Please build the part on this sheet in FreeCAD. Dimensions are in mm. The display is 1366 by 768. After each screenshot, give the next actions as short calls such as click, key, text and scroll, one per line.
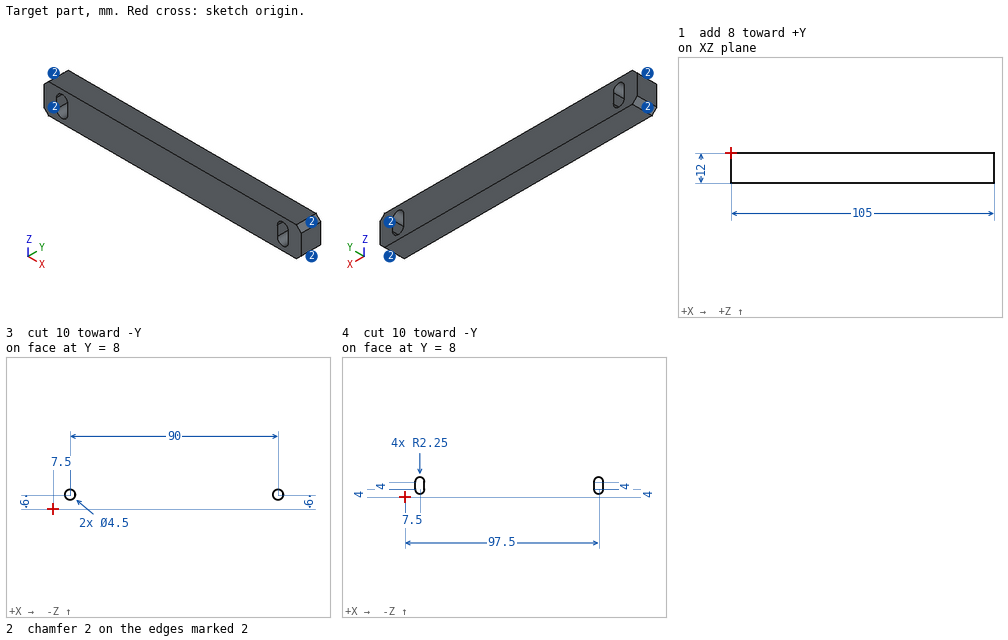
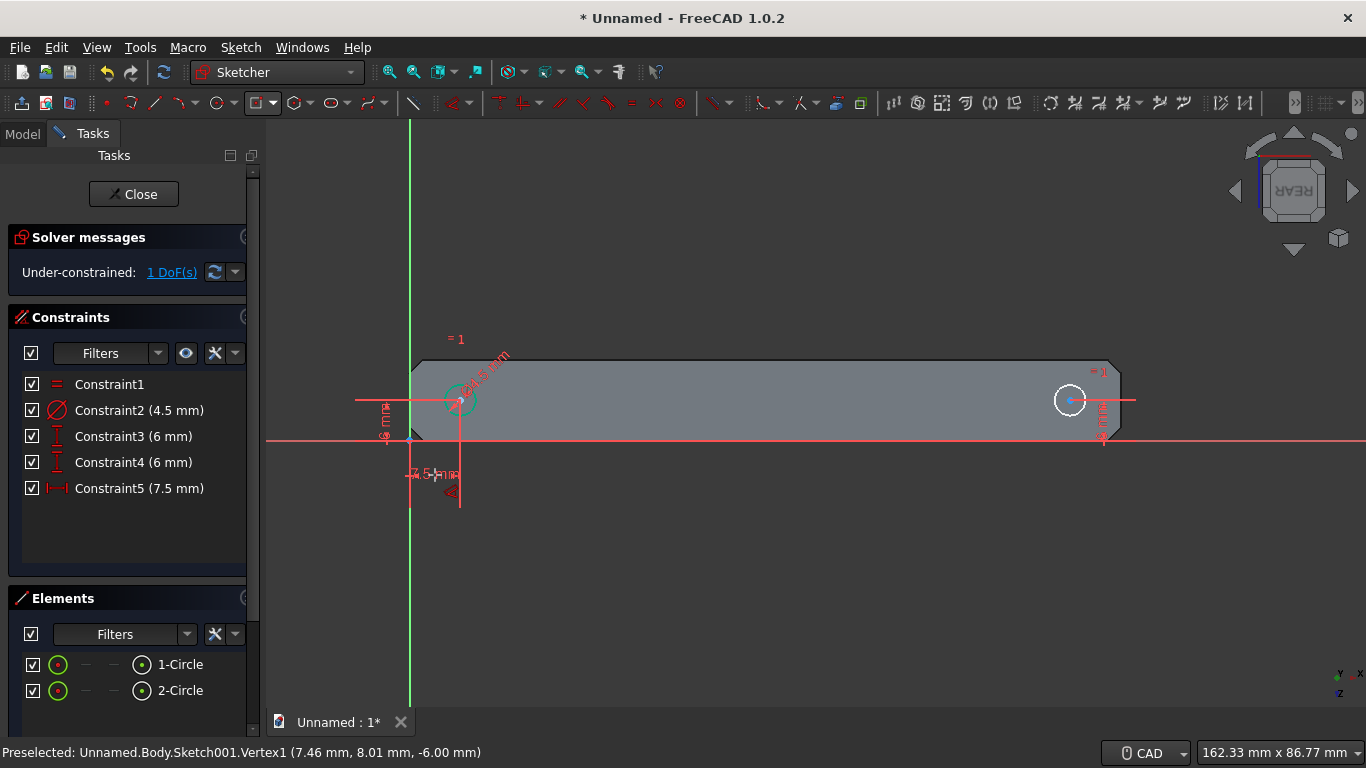
click(460, 400)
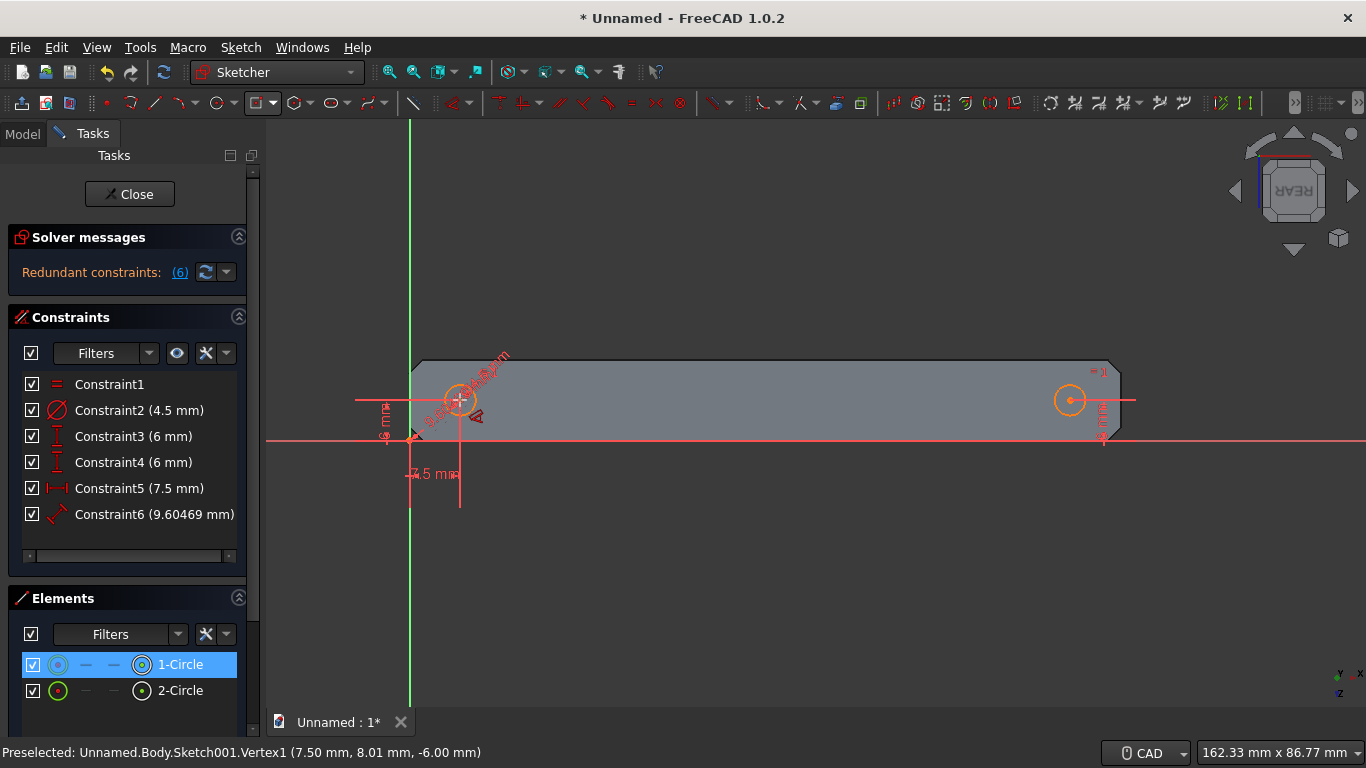
click(1070, 400)
click(765, 366)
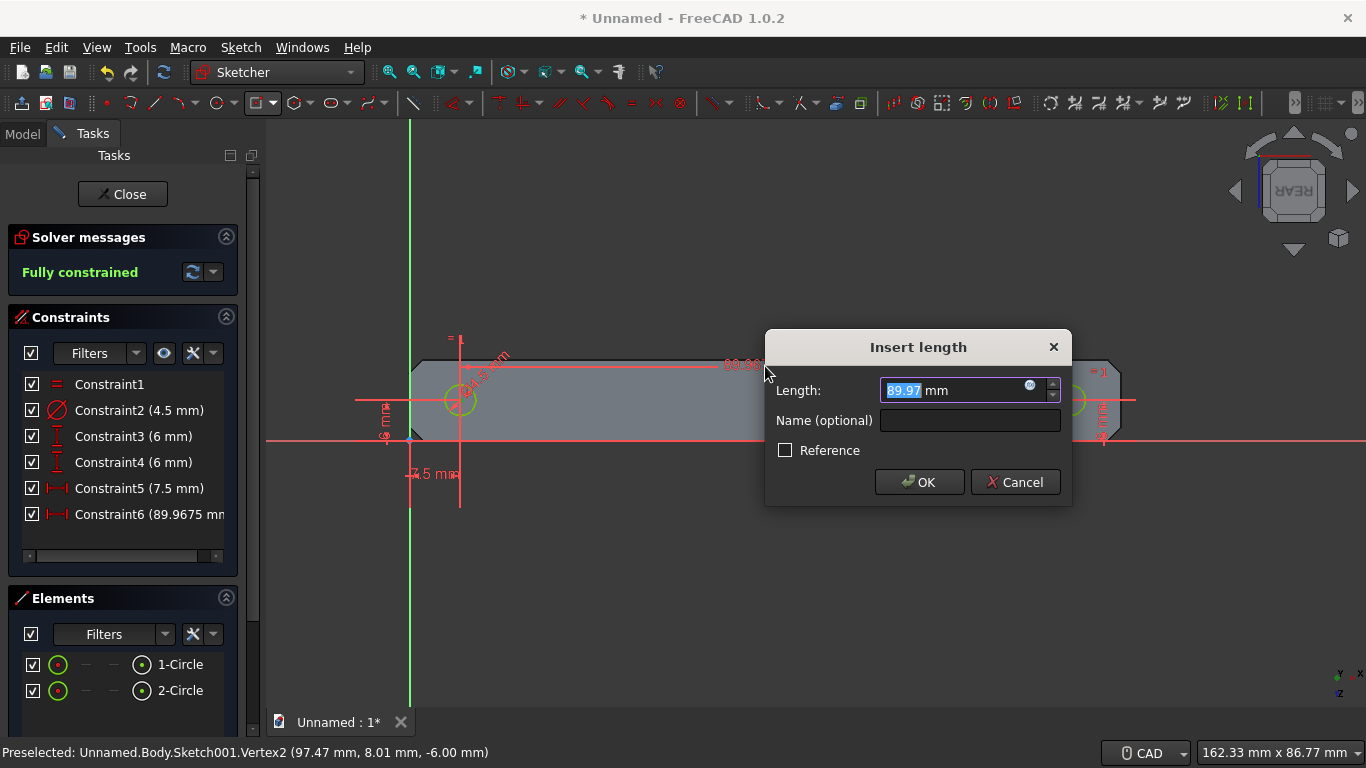
text(90)
key(Return)
key(Escape)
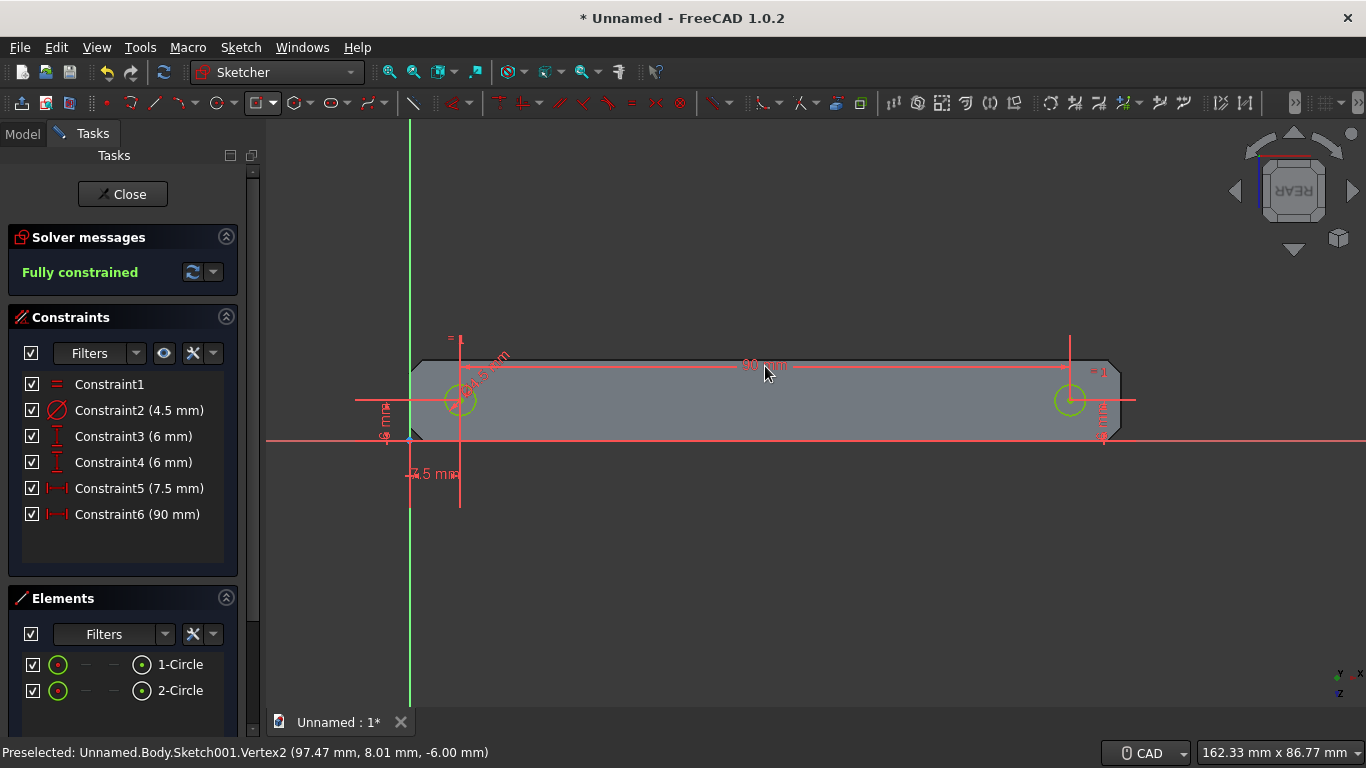
click(123, 194)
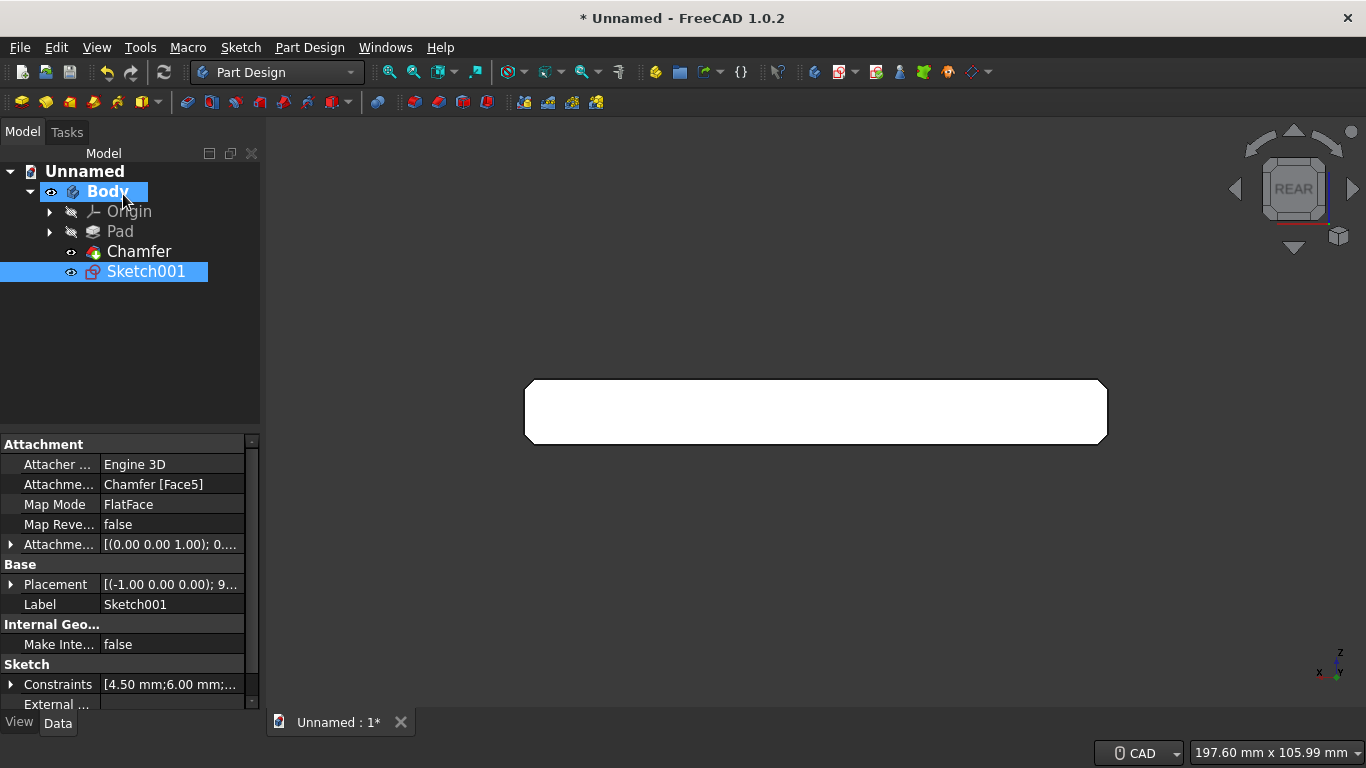
click(188, 102)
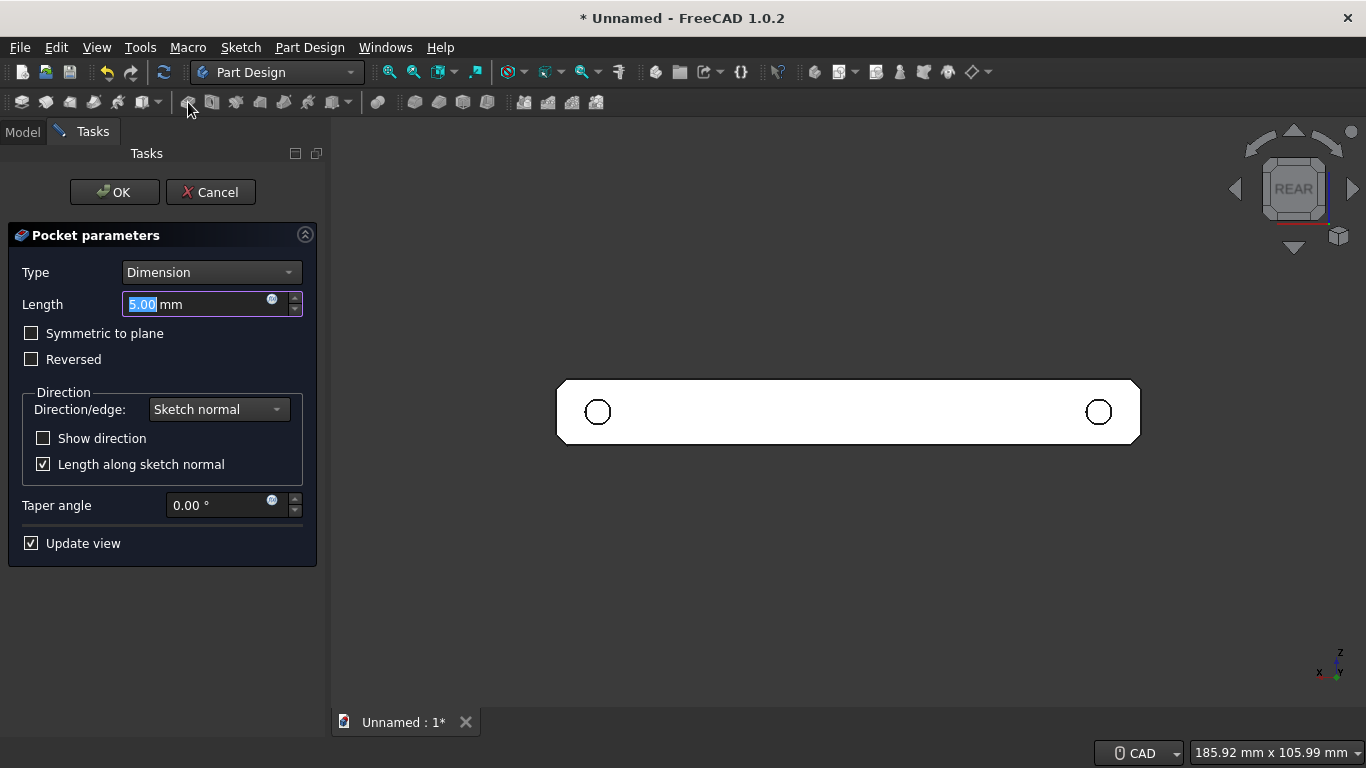
text(10)
key(Tab)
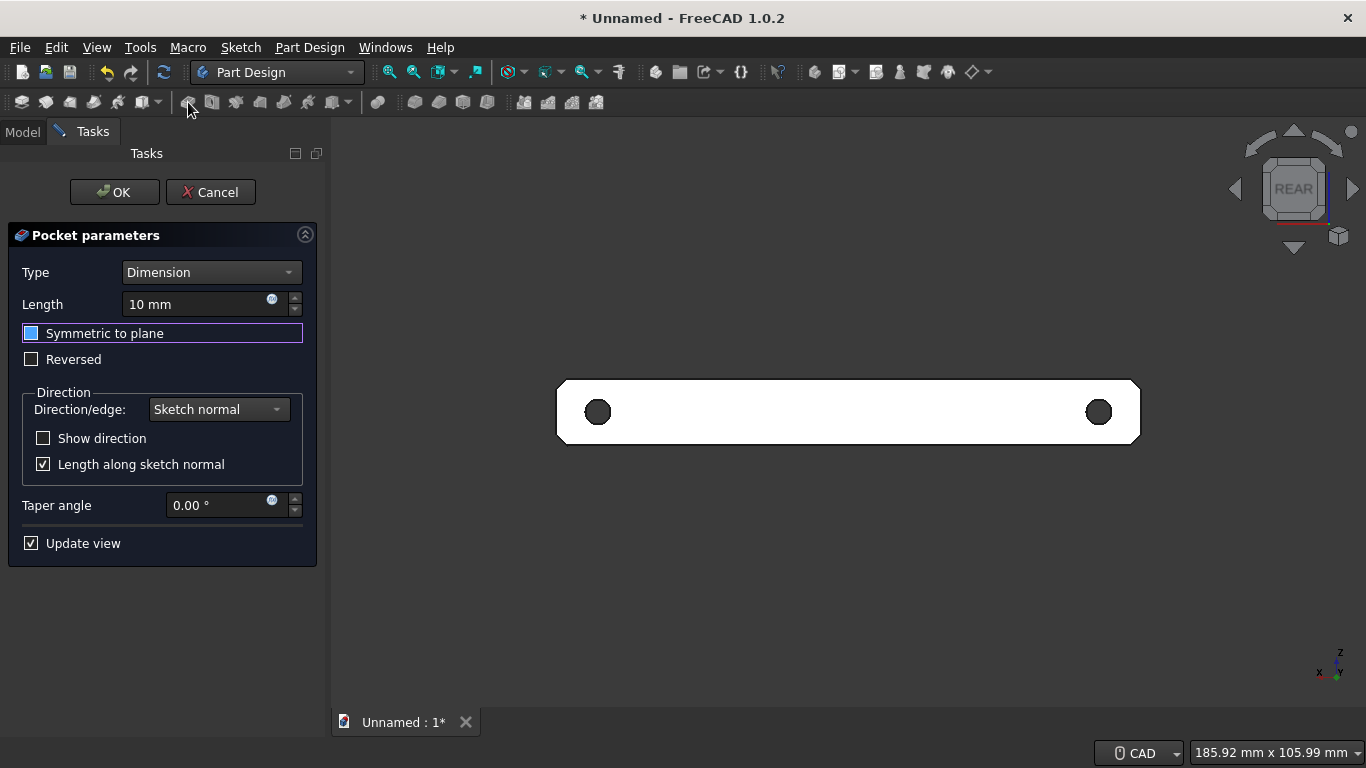
click(115, 192)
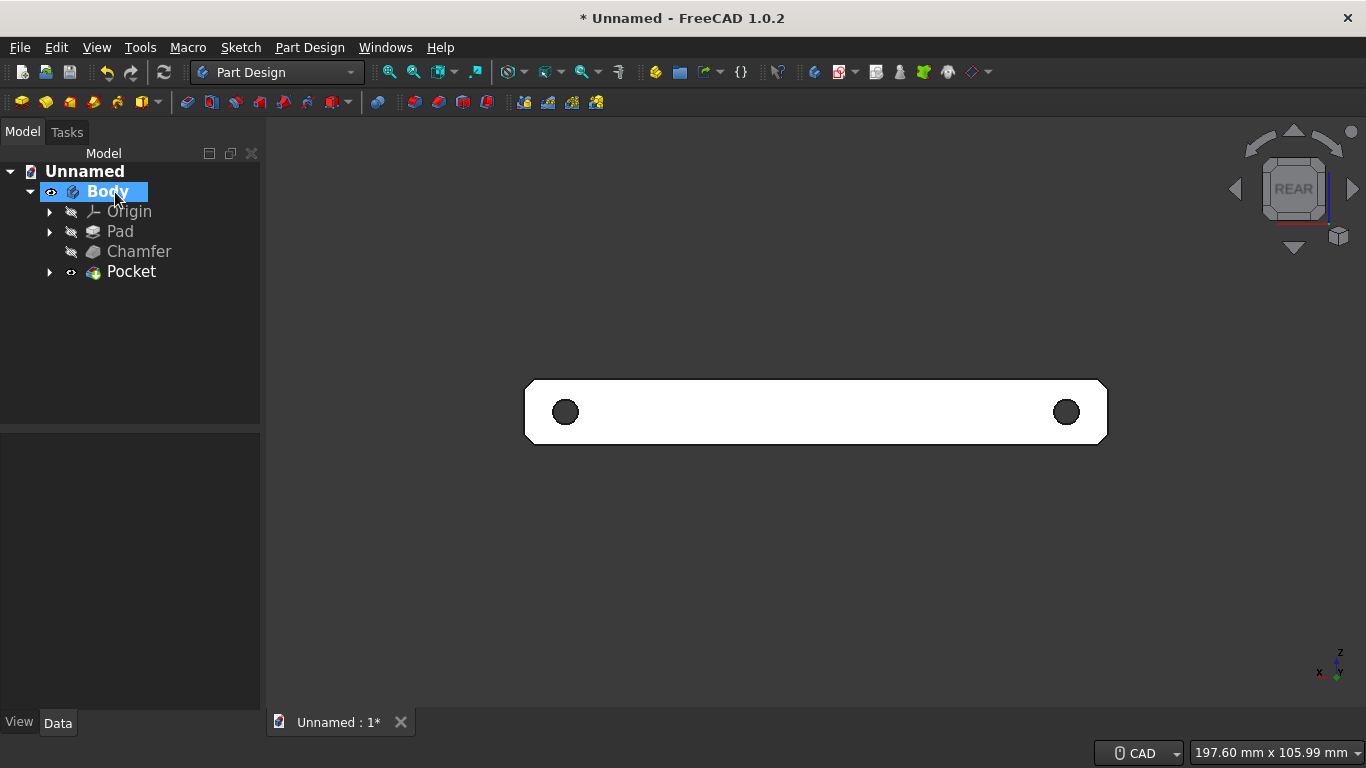
click(649, 411)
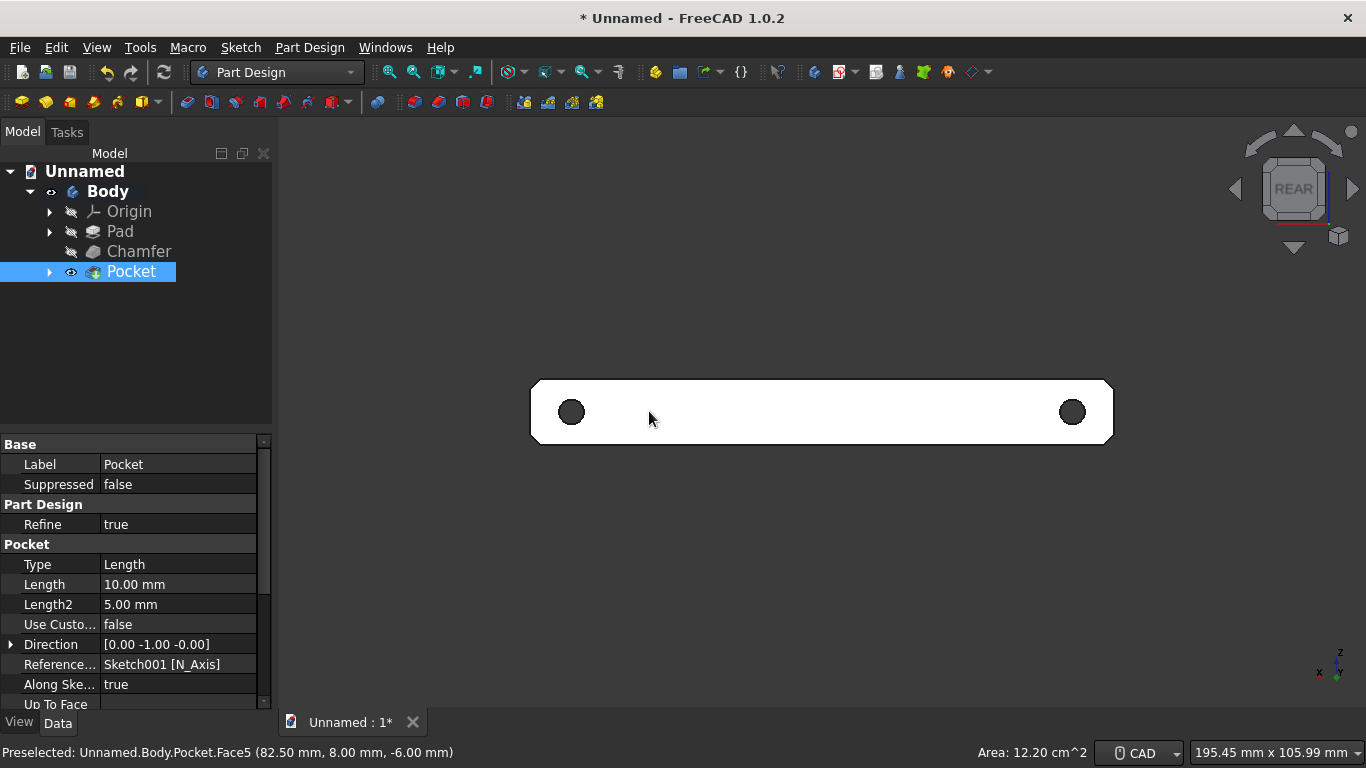
click(840, 72)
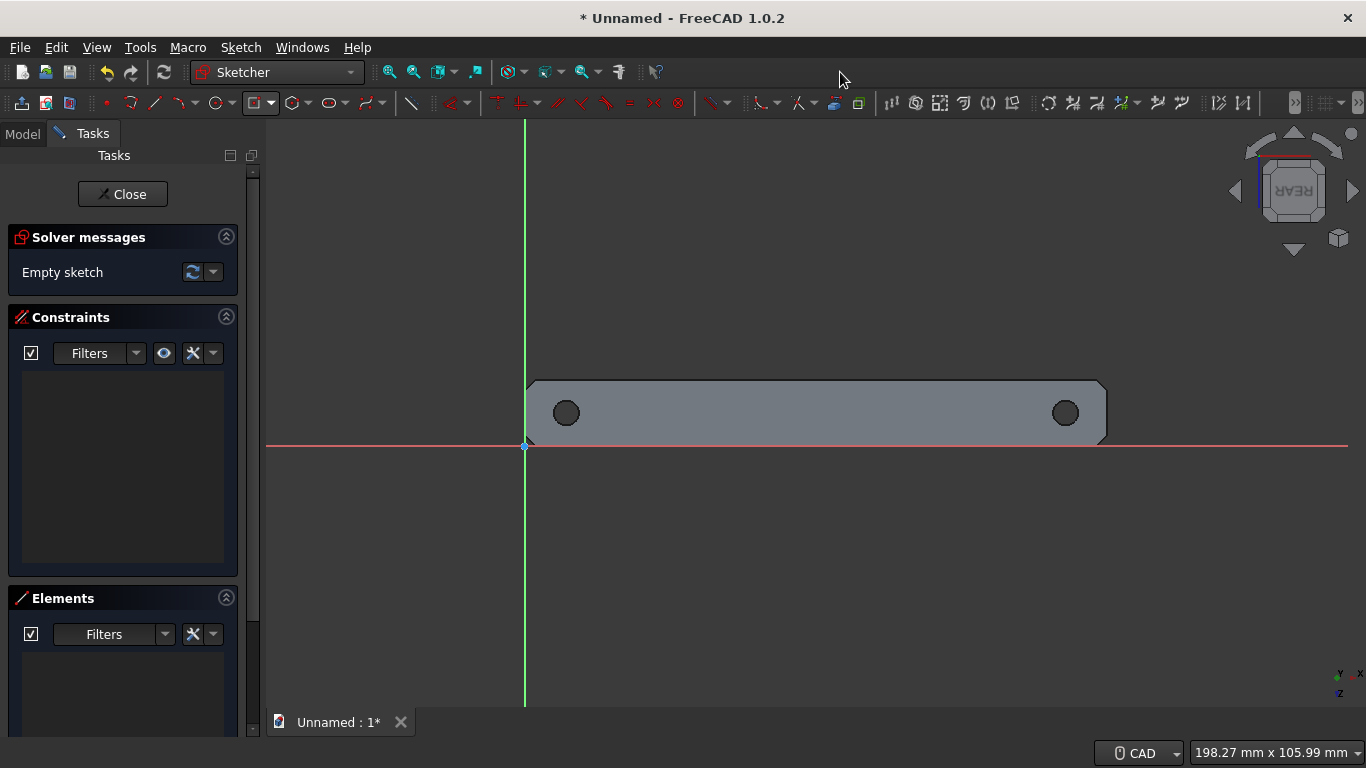
click(330, 104)